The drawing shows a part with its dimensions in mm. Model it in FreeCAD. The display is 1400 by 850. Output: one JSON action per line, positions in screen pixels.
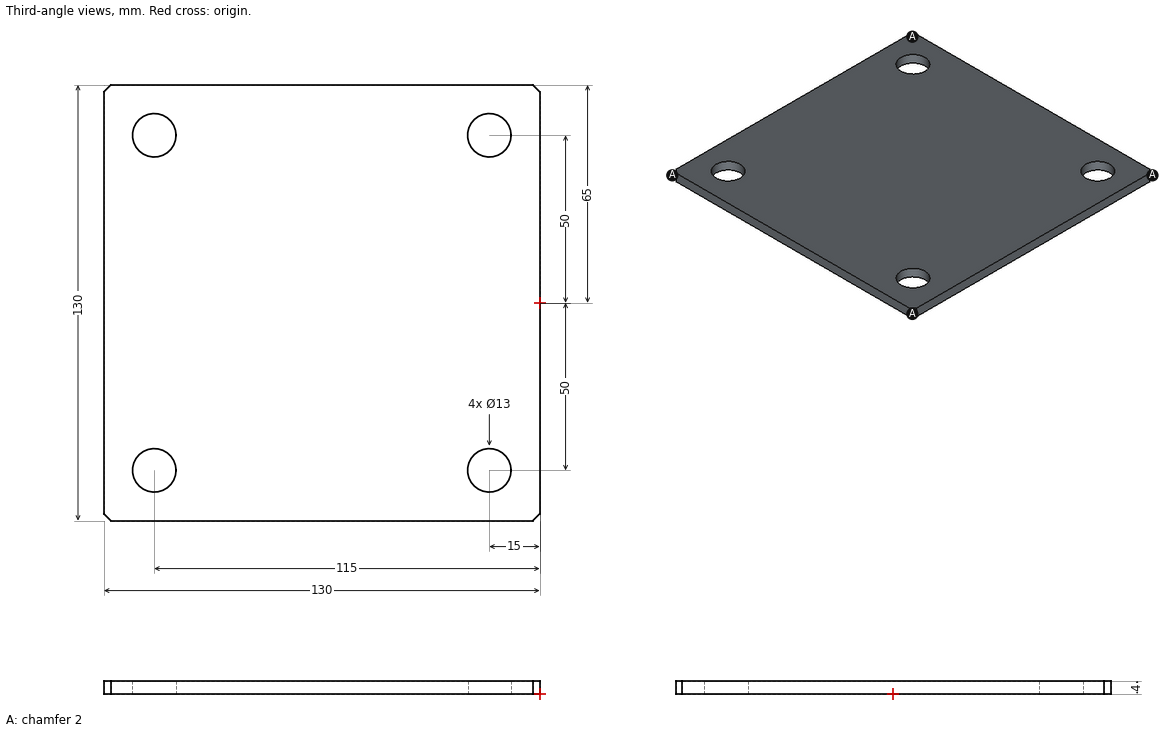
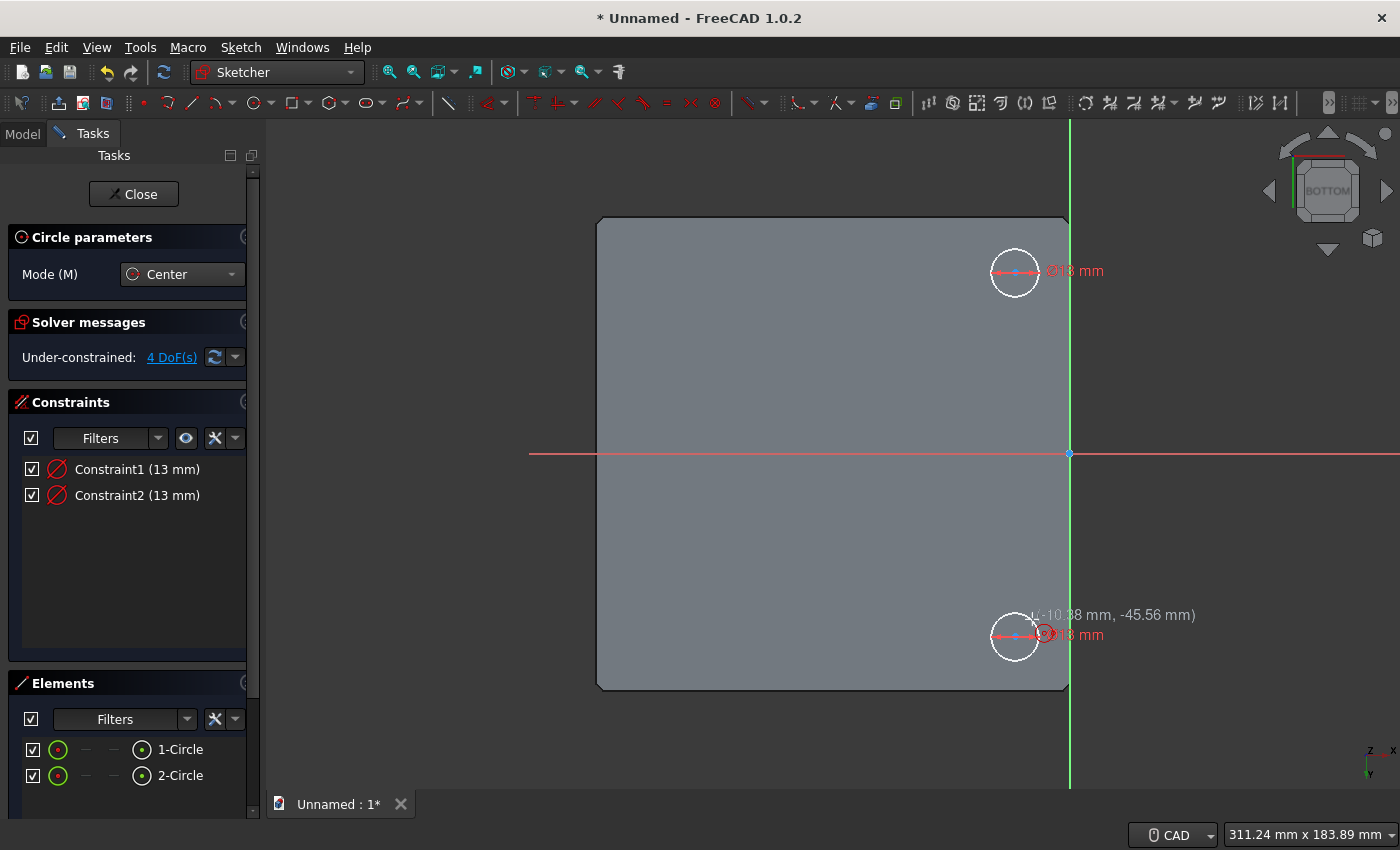
{"action": "left_click", "coordinate": [651, 272]}
{"action": "mouse_move", "coordinate": [668, 255]}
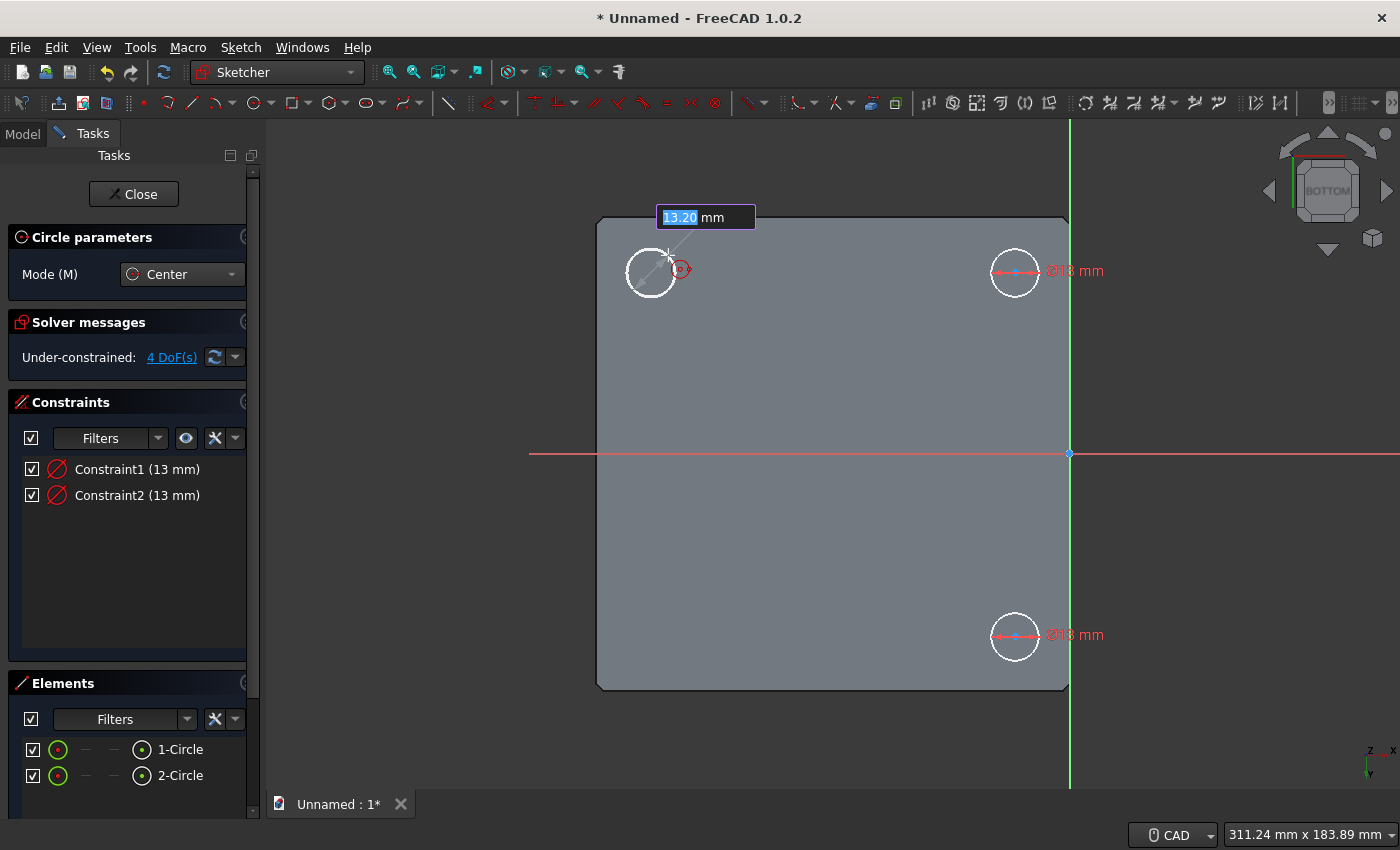
{"action": "type", "text": "13"}
{"action": "key", "text": "Return"}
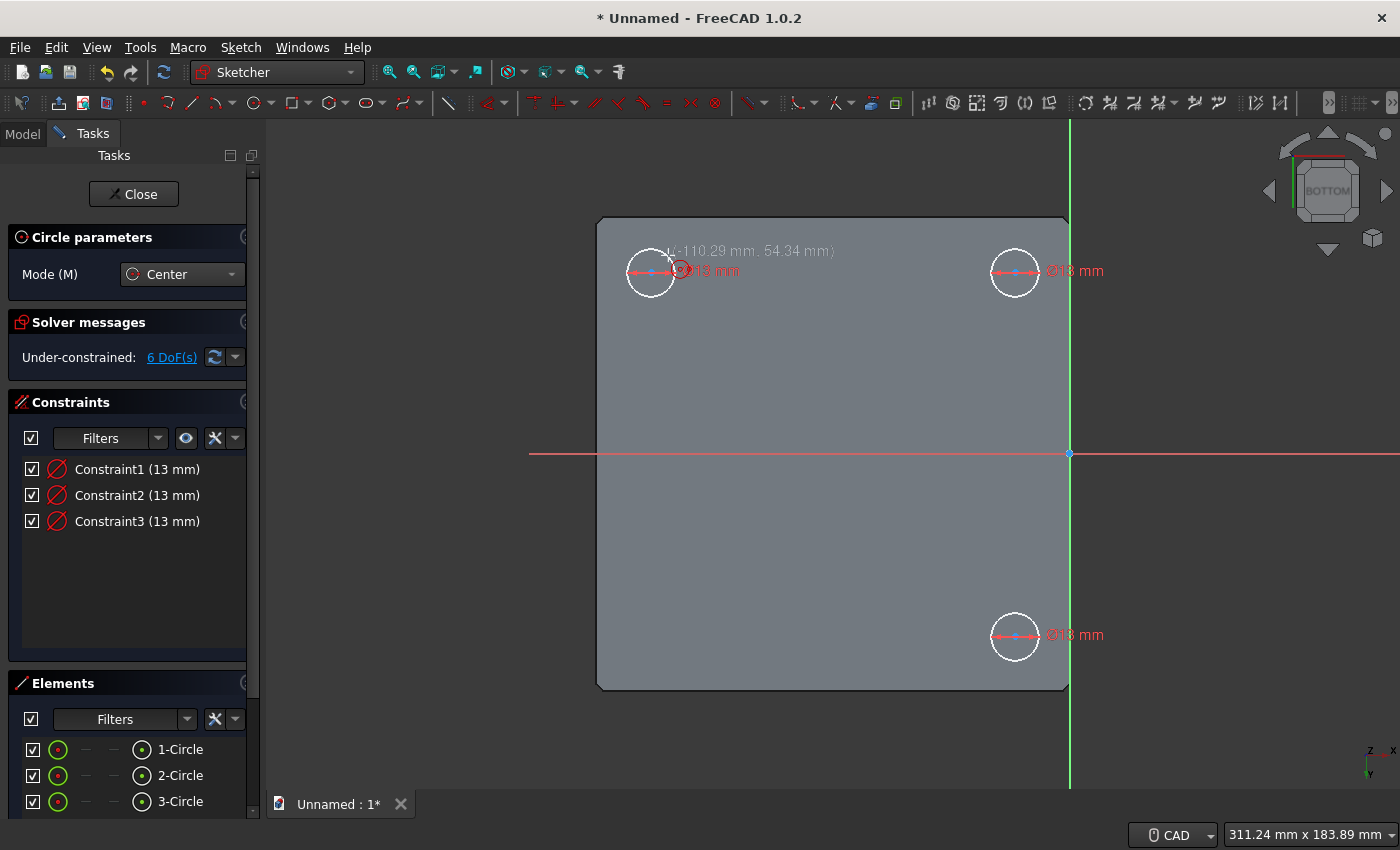
{"action": "left_click", "coordinate": [651, 636]}
{"action": "mouse_move", "coordinate": [668, 619]}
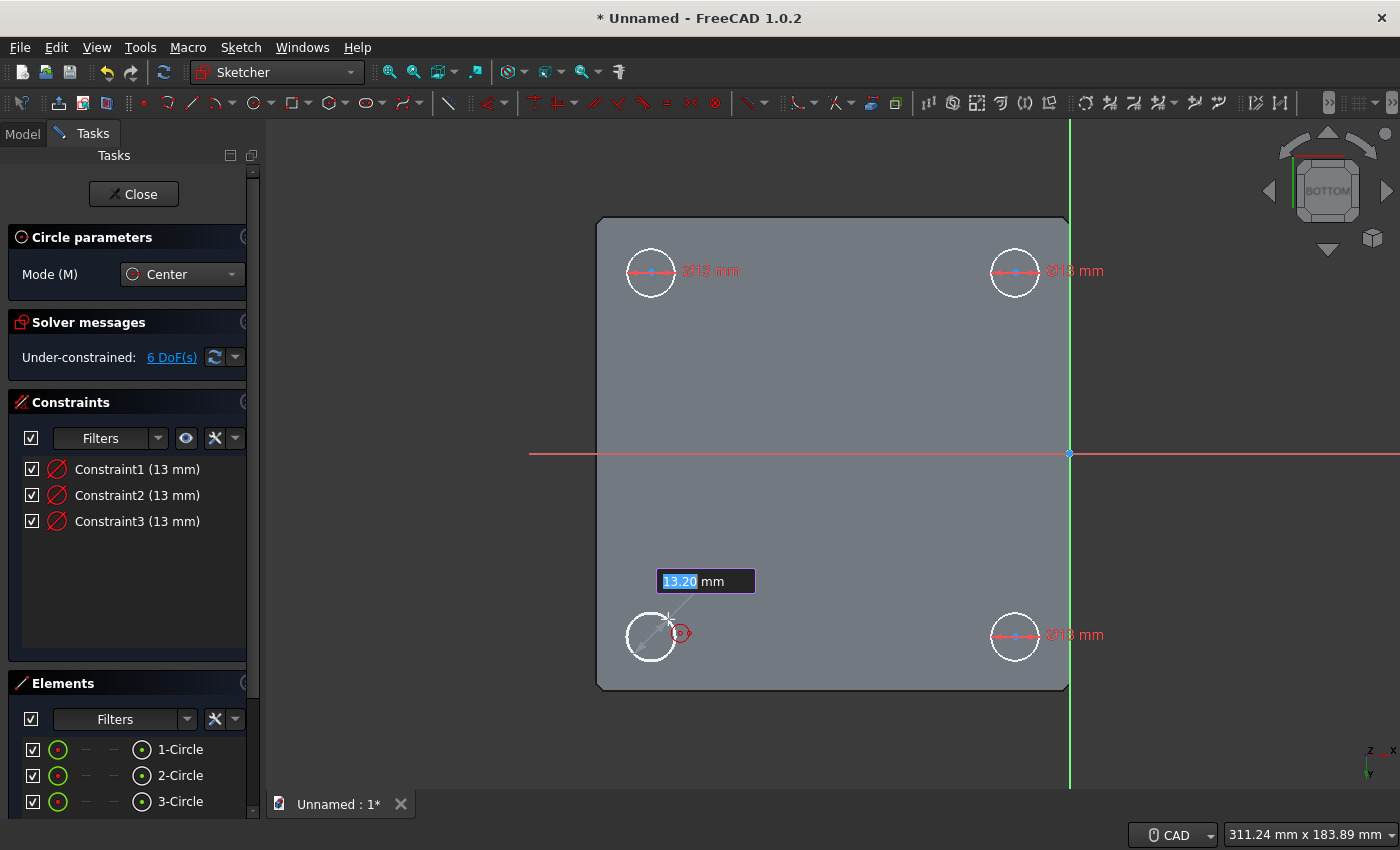
{"action": "type", "text": "13"}
{"action": "key", "text": "Return"}
{"action": "key", "text": "Escape"}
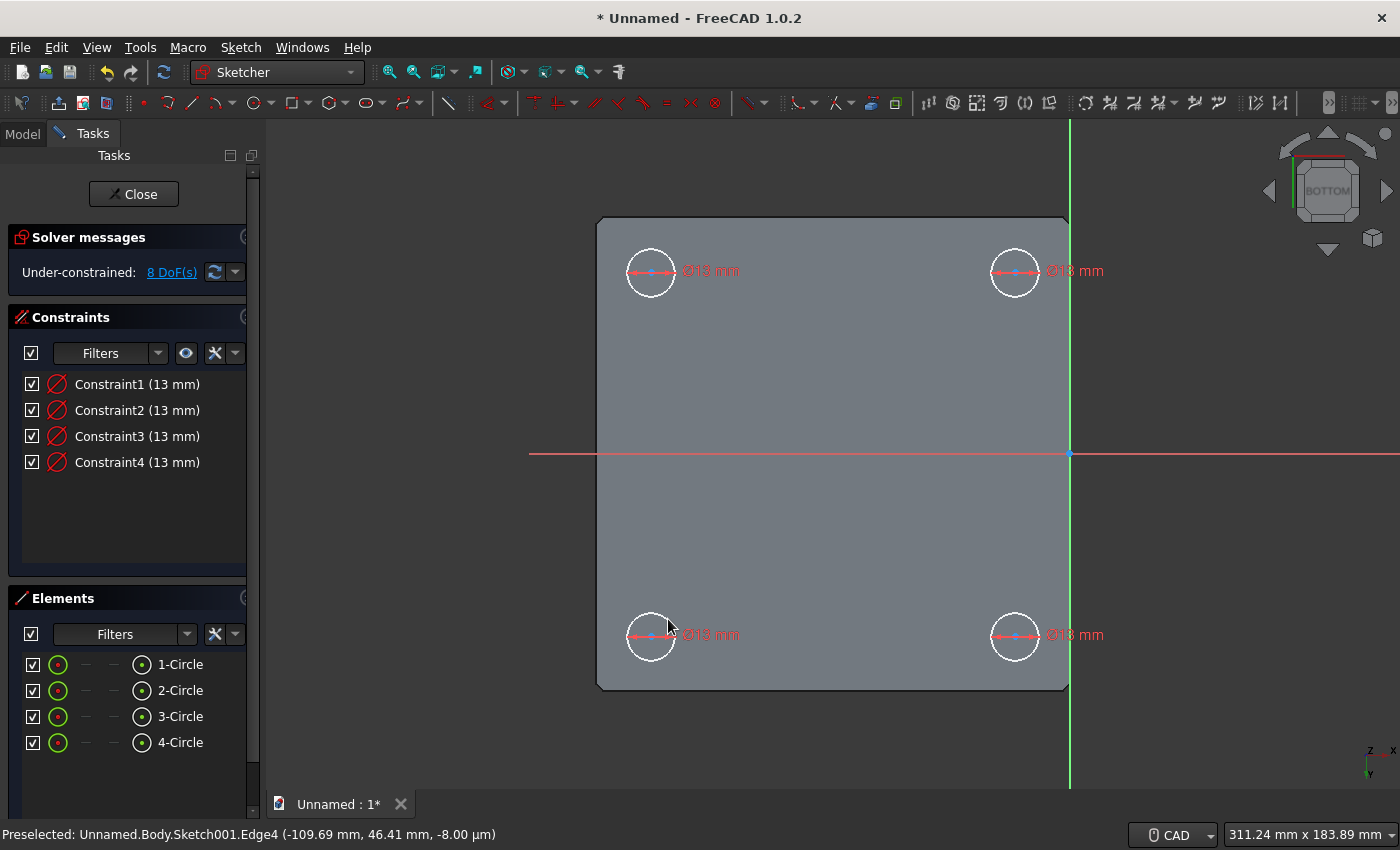
{"action": "left_click", "coordinate": [488, 104]}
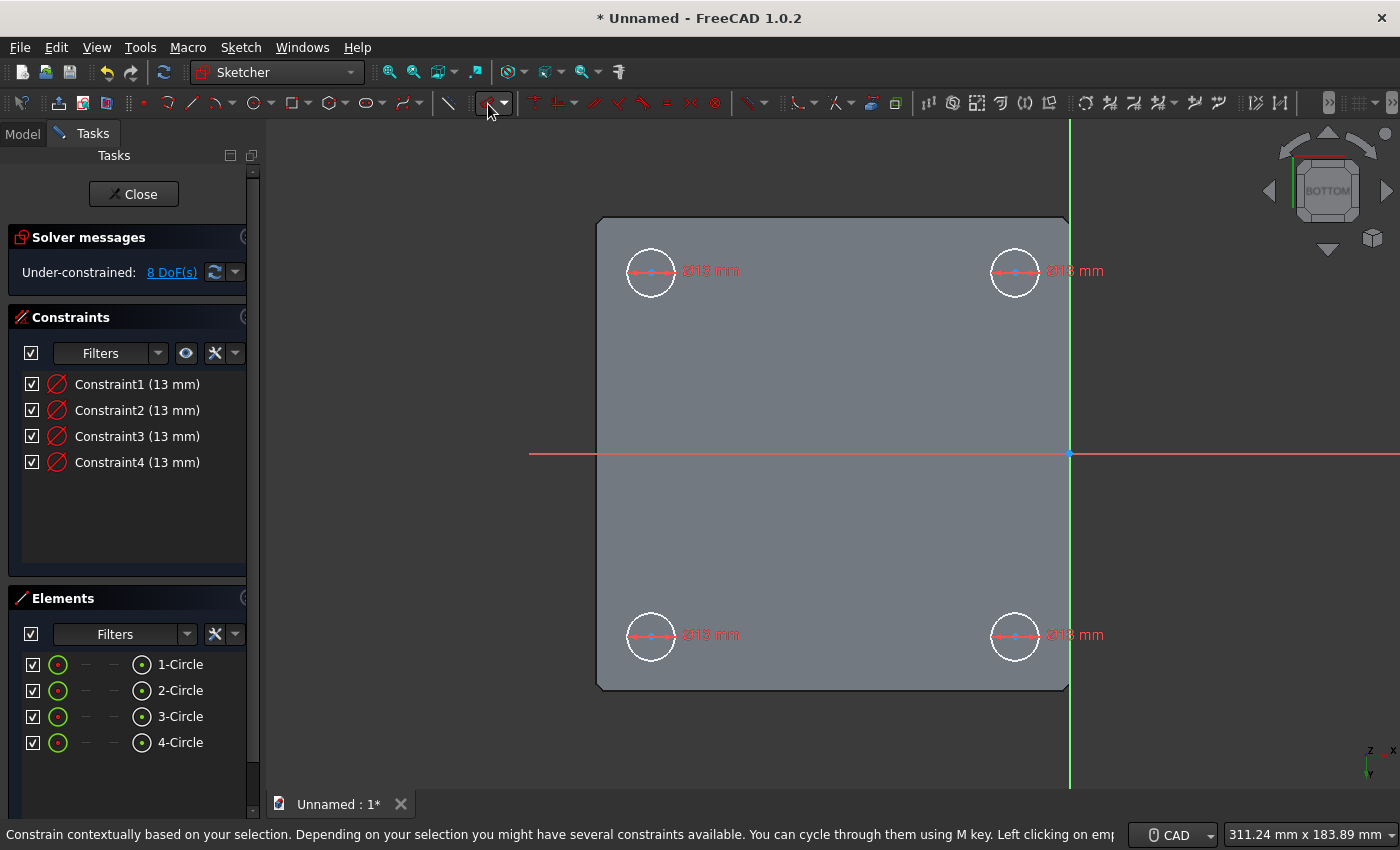
{"action": "left_click", "coordinate": [1015, 273]}
{"action": "left_click", "coordinate": [1042, 239]}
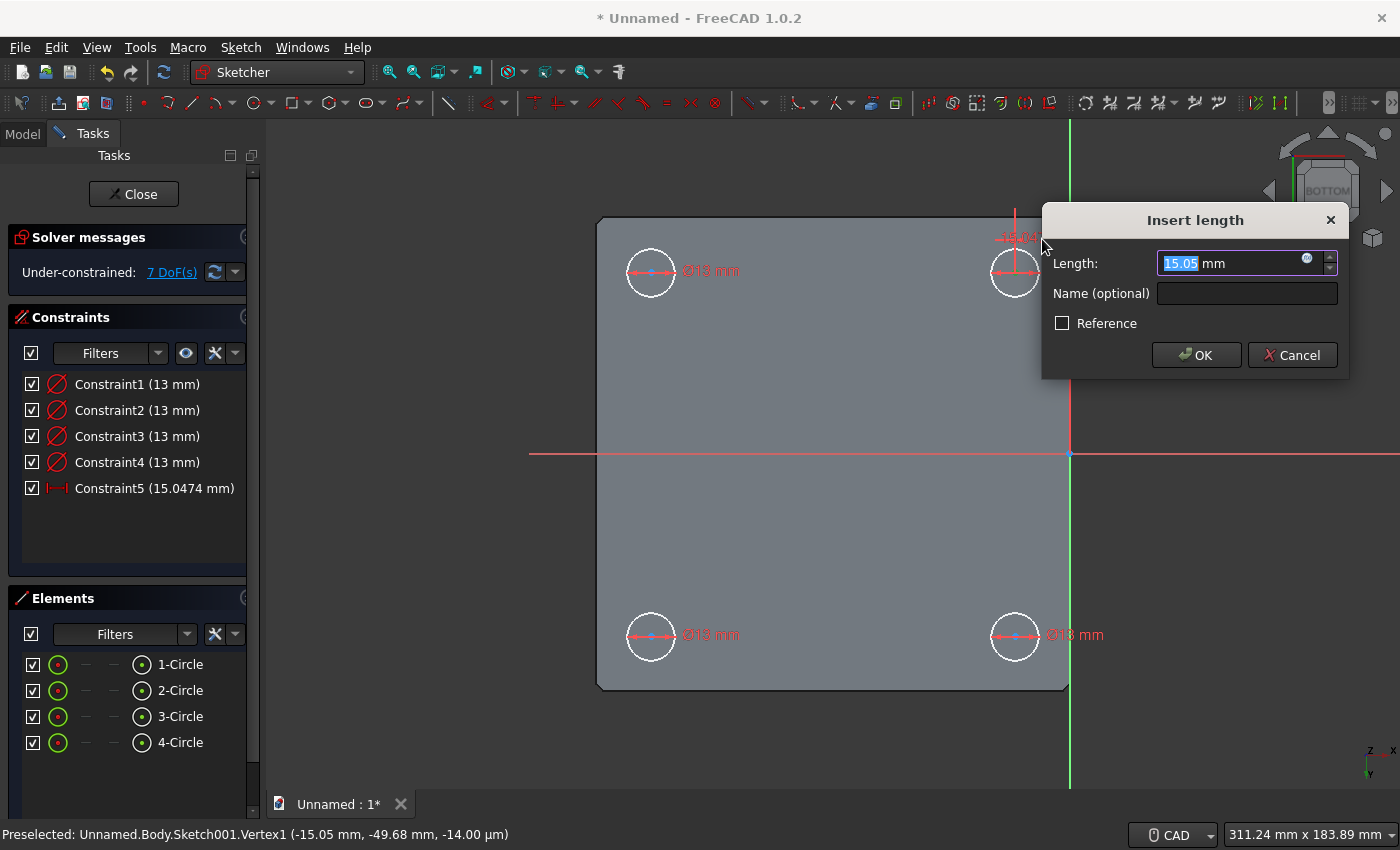
{"action": "type", "text": "15"}
{"action": "key", "text": "Return"}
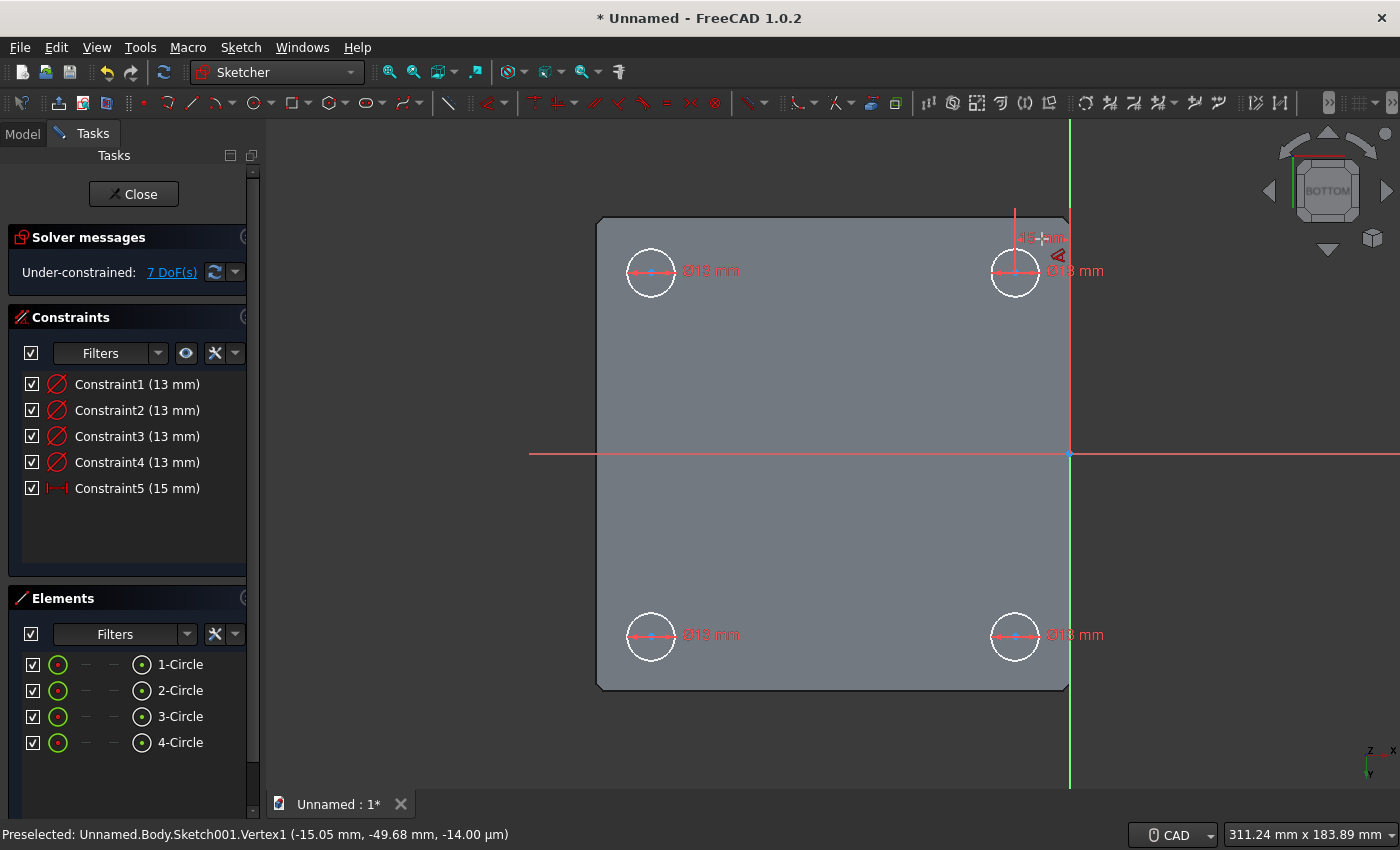
{"action": "left_click", "coordinate": [1015, 273]}
{"action": "left_click", "coordinate": [1104, 364]}